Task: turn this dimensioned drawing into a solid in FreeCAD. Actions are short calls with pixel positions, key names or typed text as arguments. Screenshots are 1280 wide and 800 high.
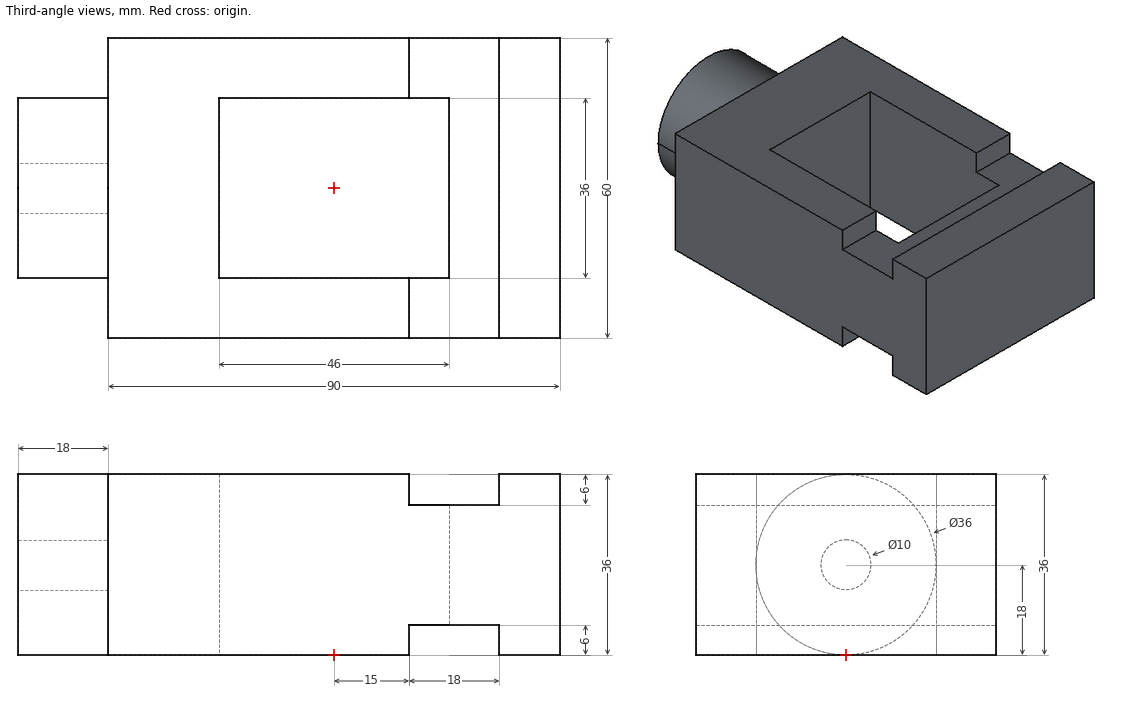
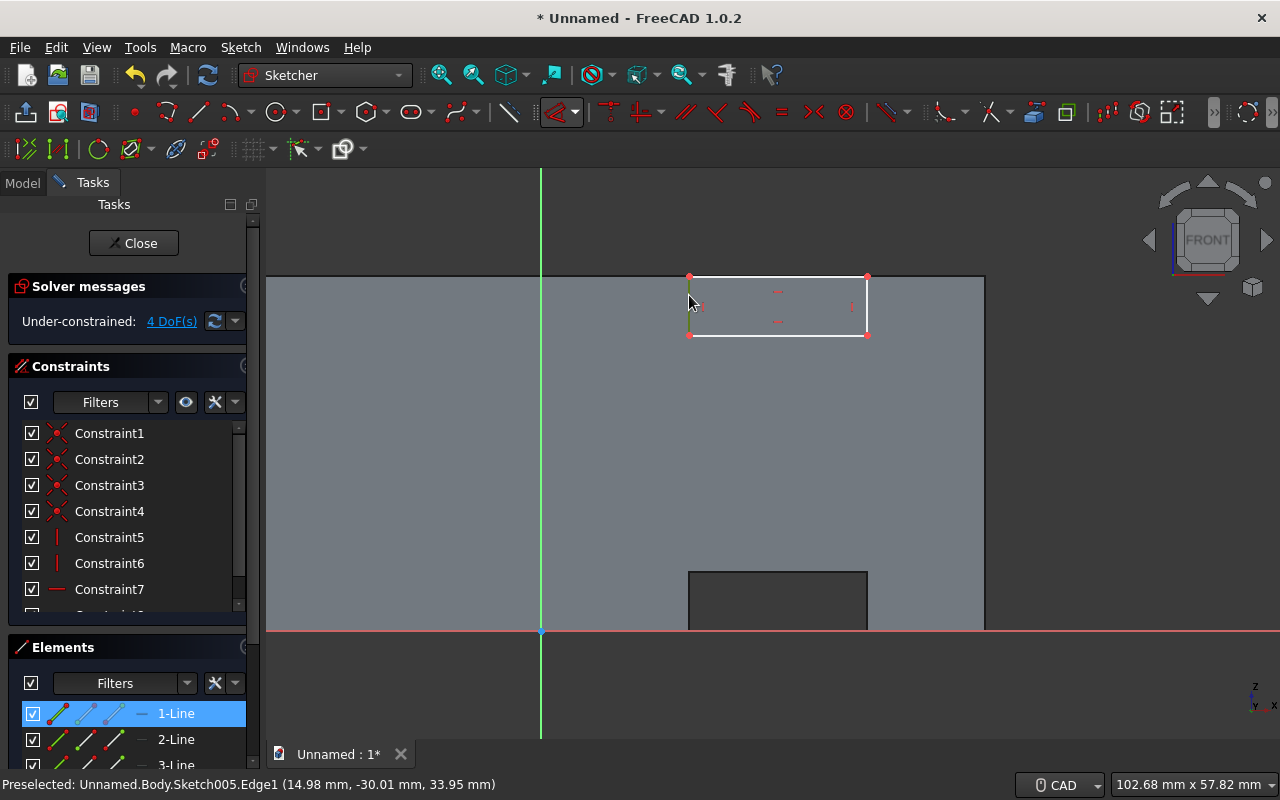
key(i)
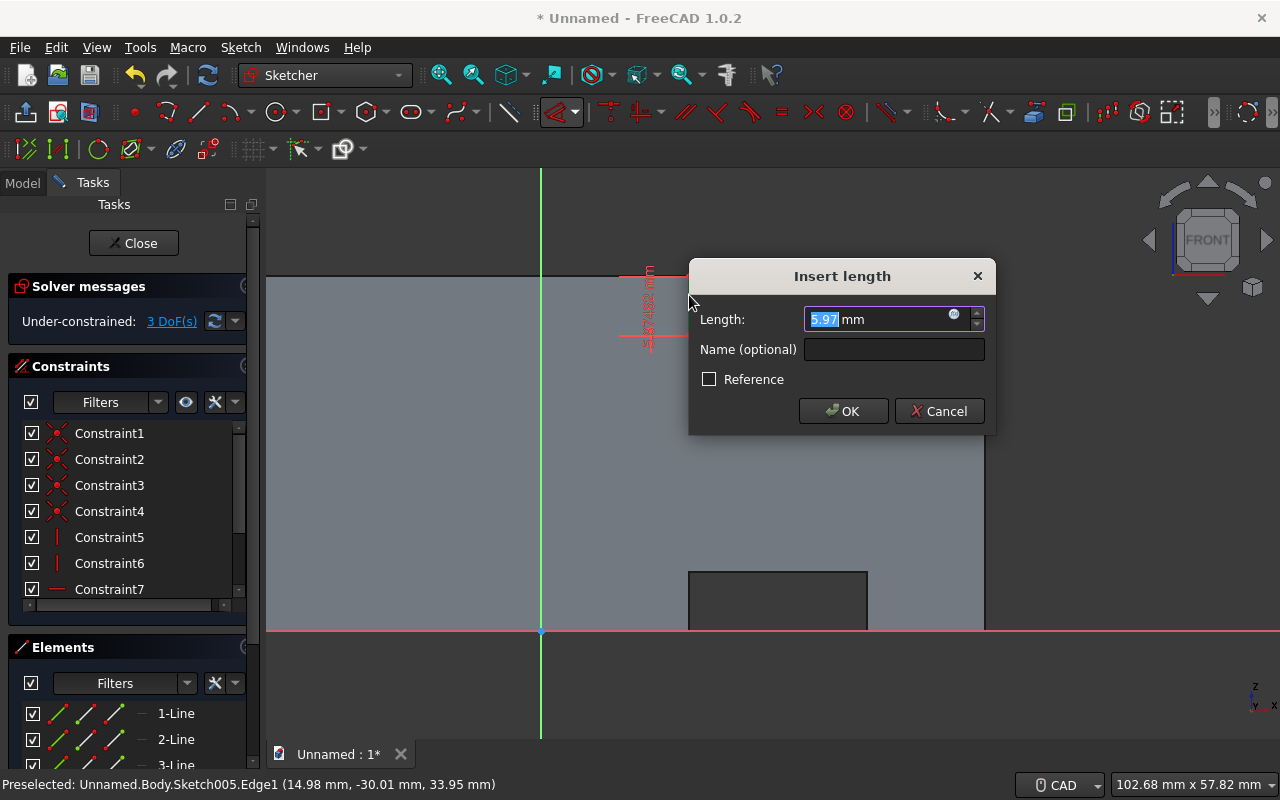
text(6)
key(Return)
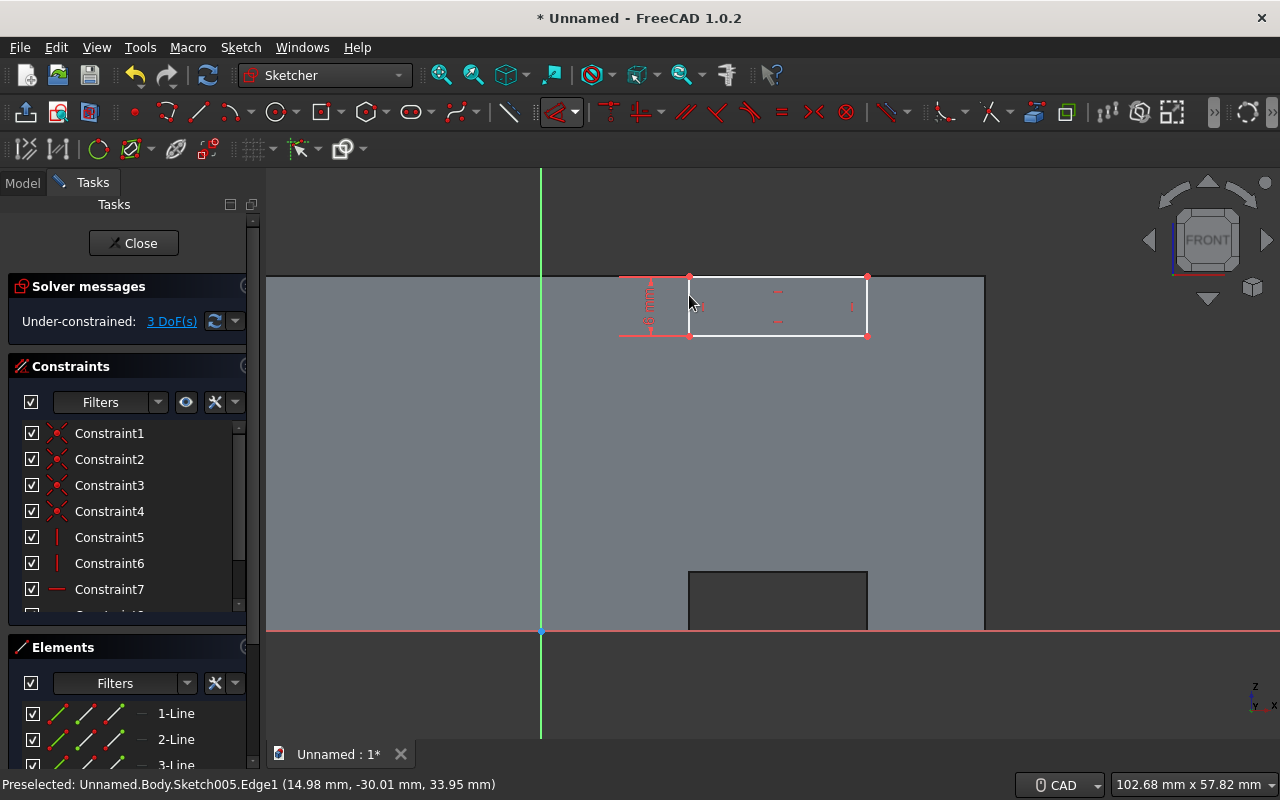
click(742, 336)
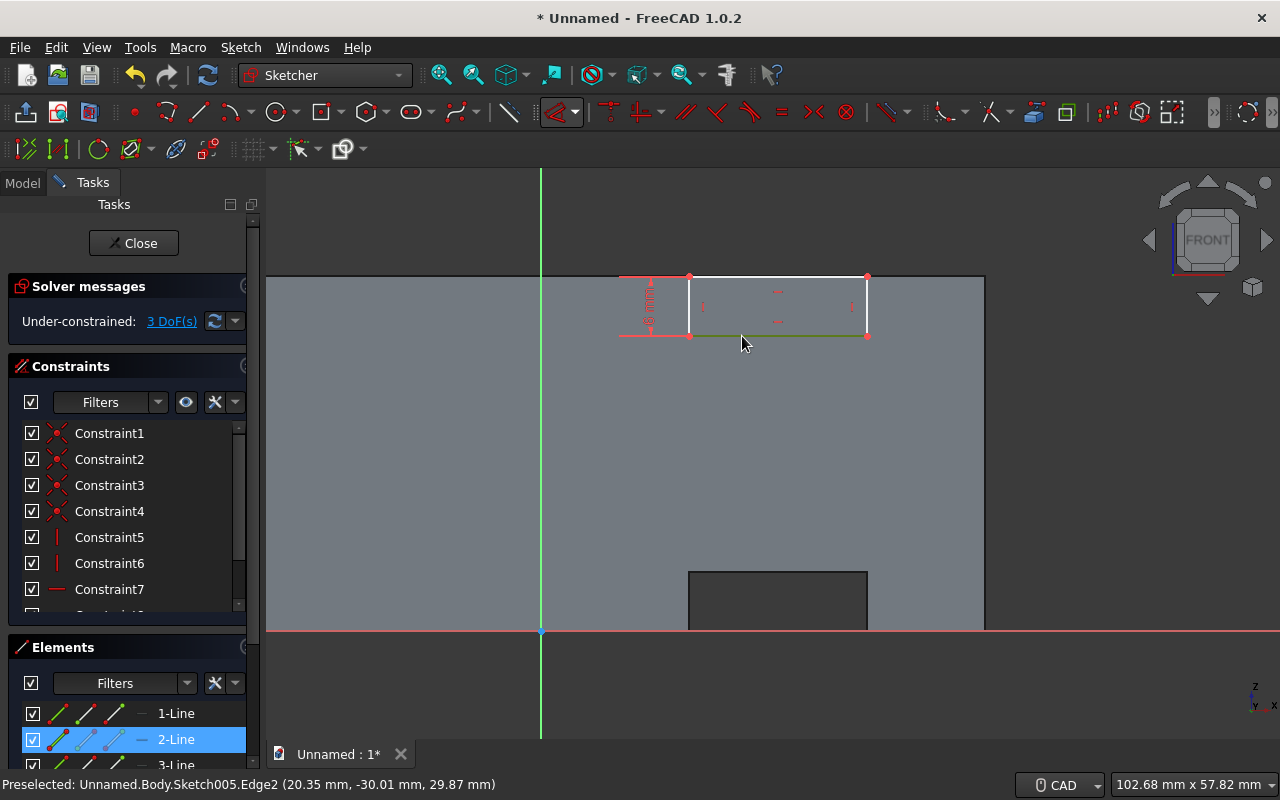
key(l)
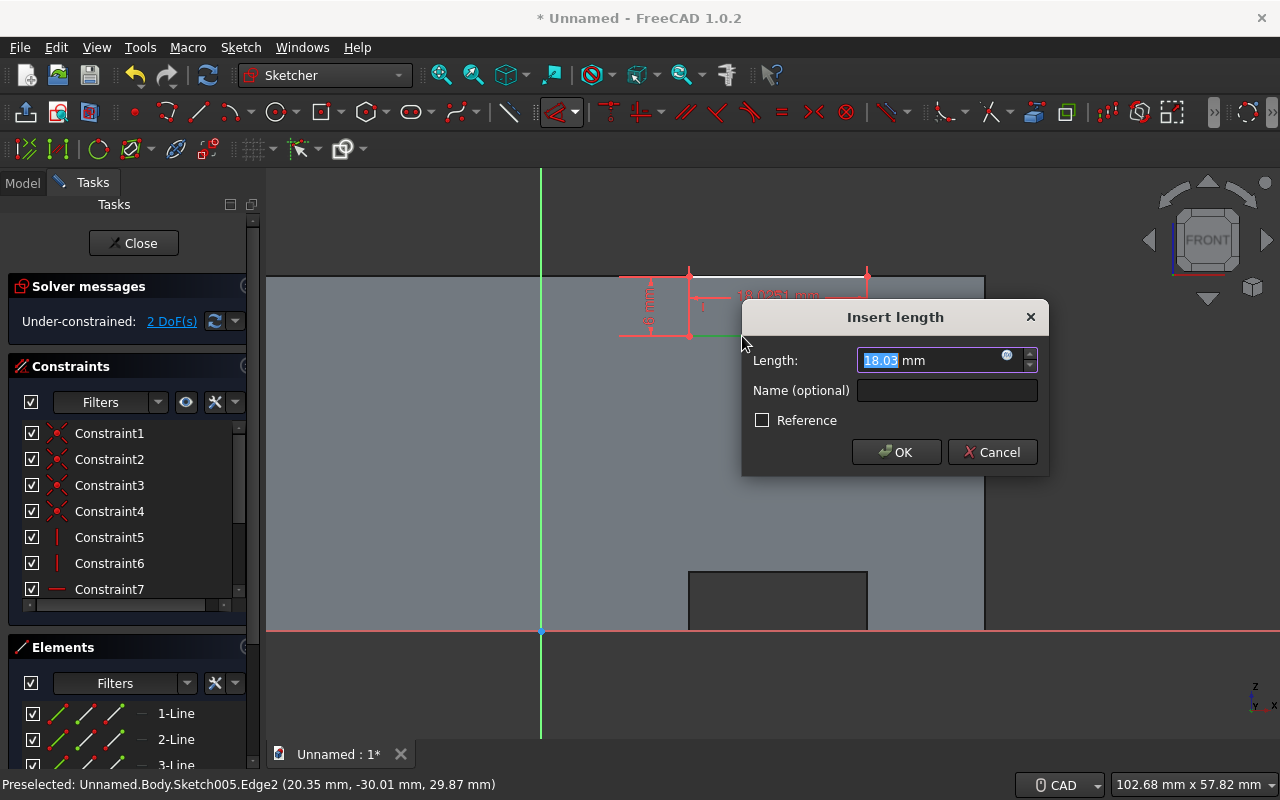
text(18)
key(Return)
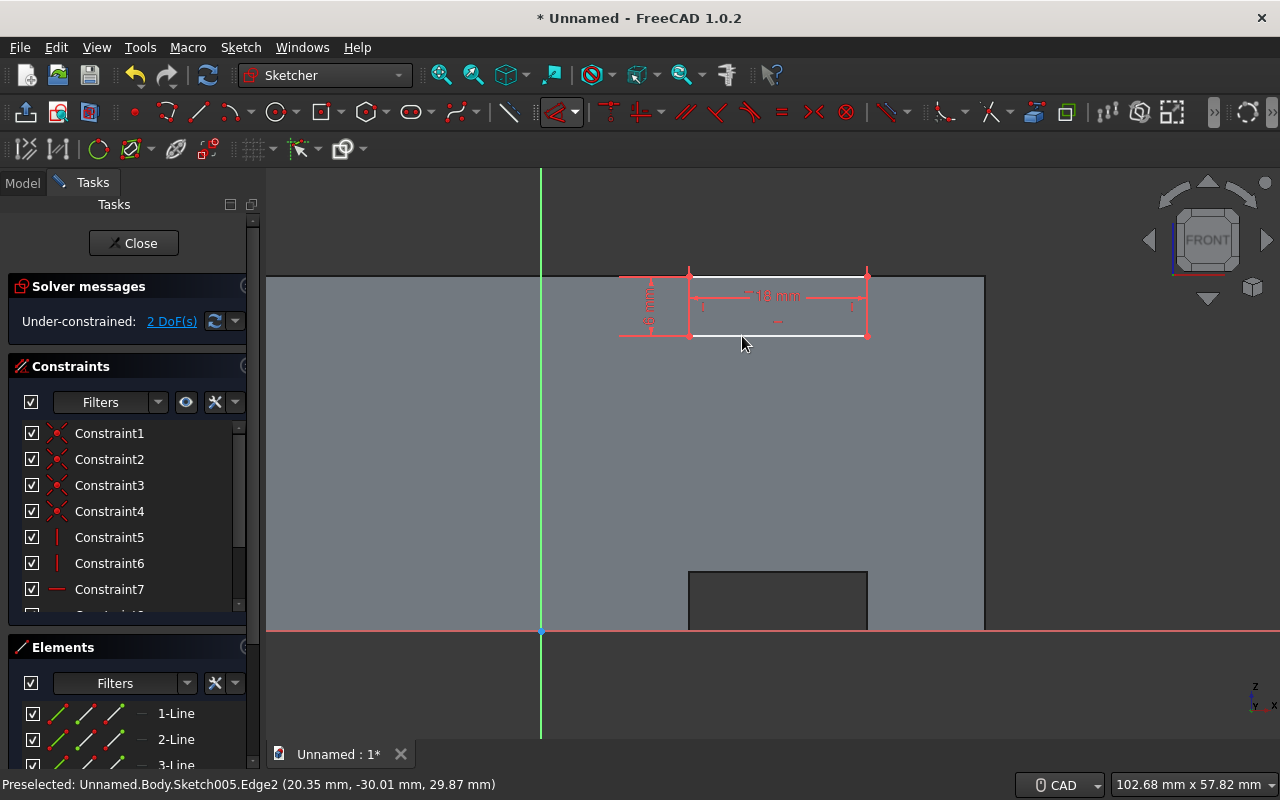
click(689, 277)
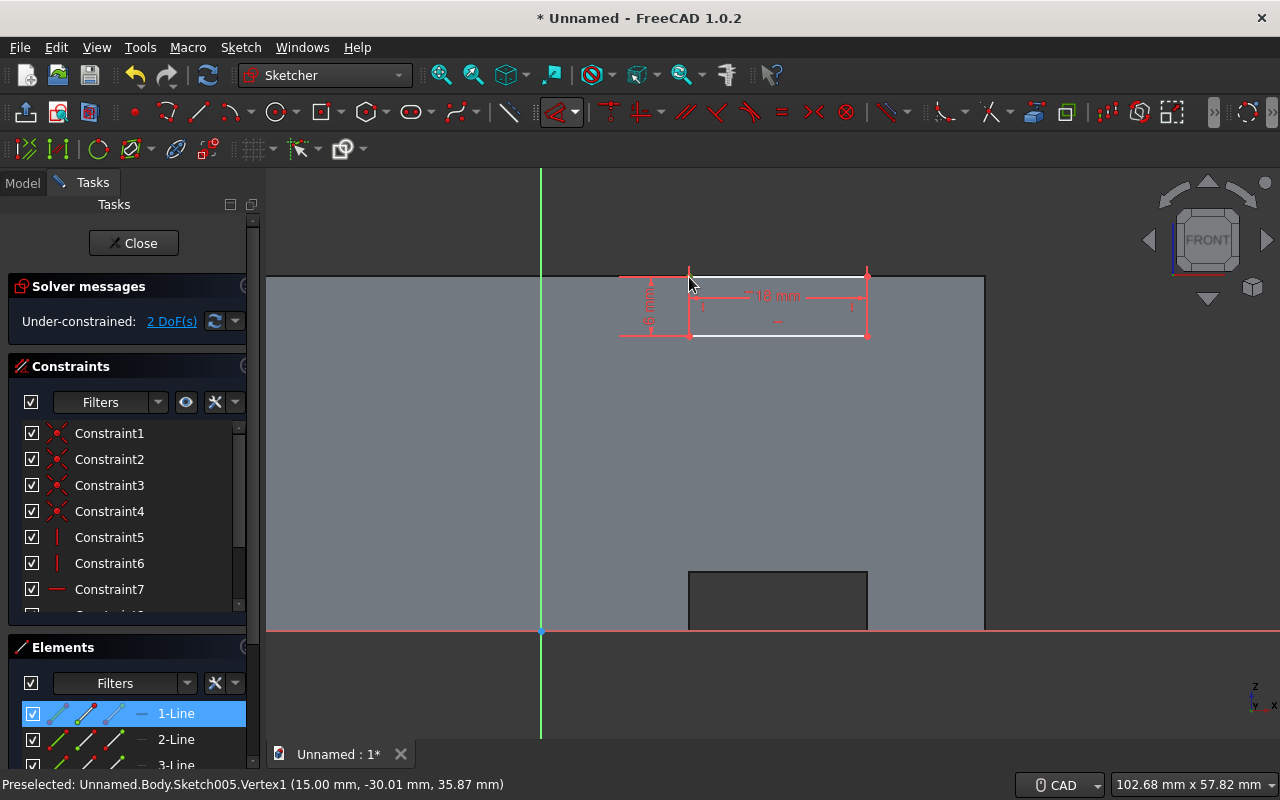
key(l)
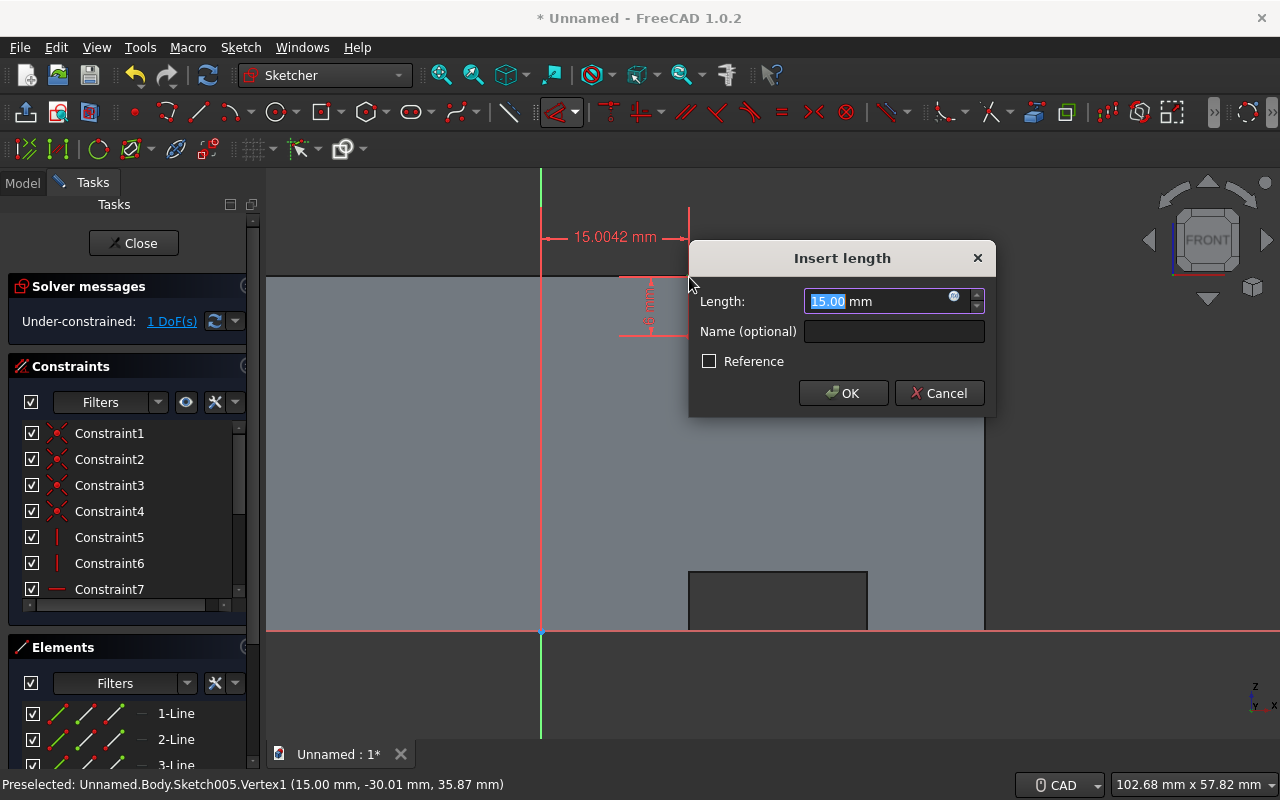
text(15)
key(Return)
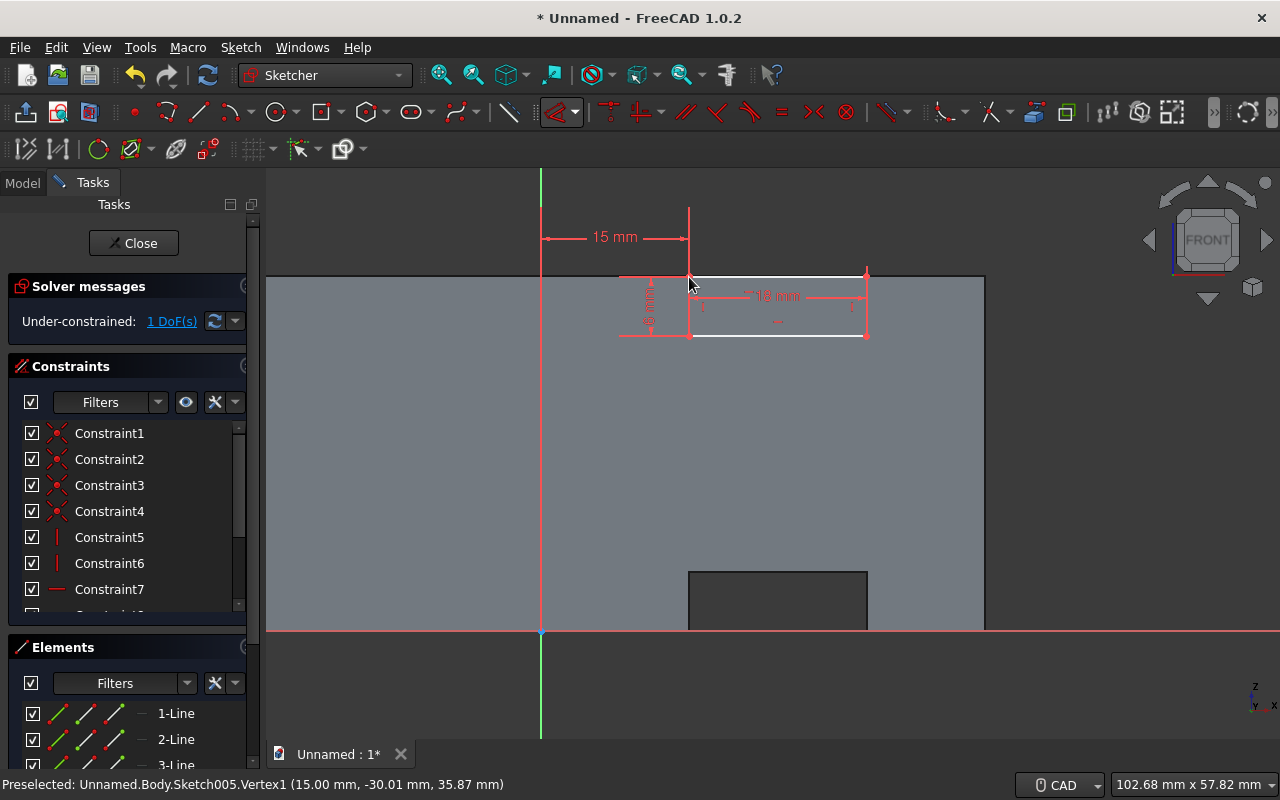
click(689, 277)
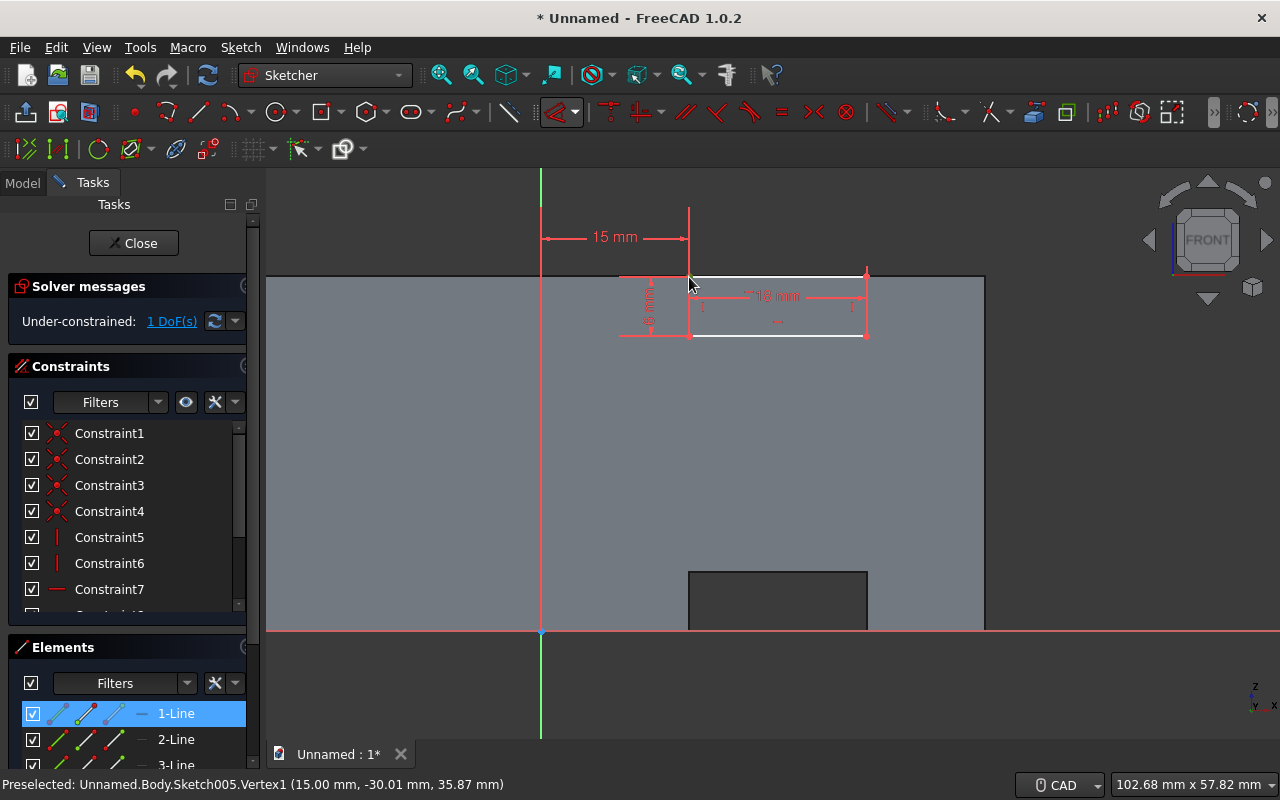
click(578, 112)